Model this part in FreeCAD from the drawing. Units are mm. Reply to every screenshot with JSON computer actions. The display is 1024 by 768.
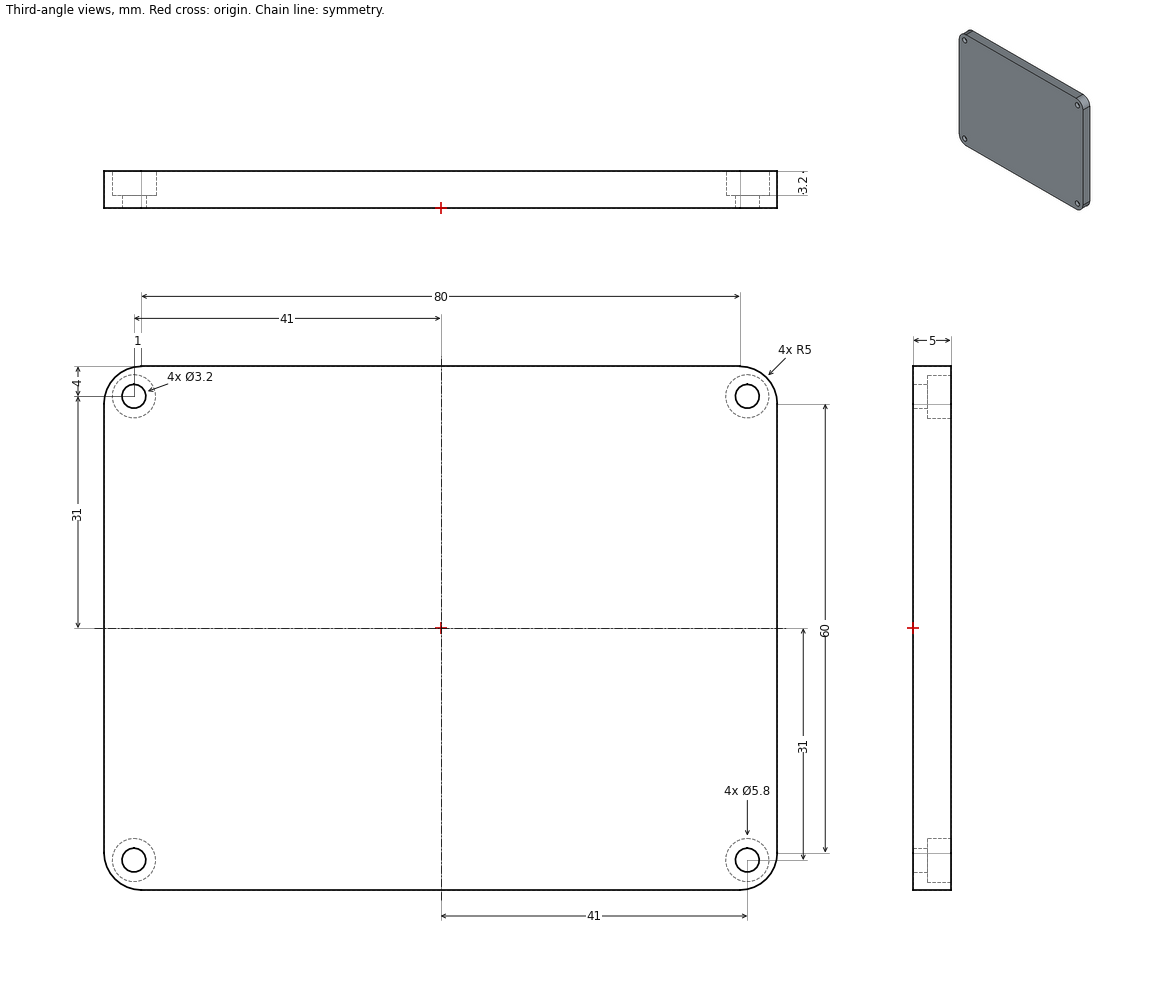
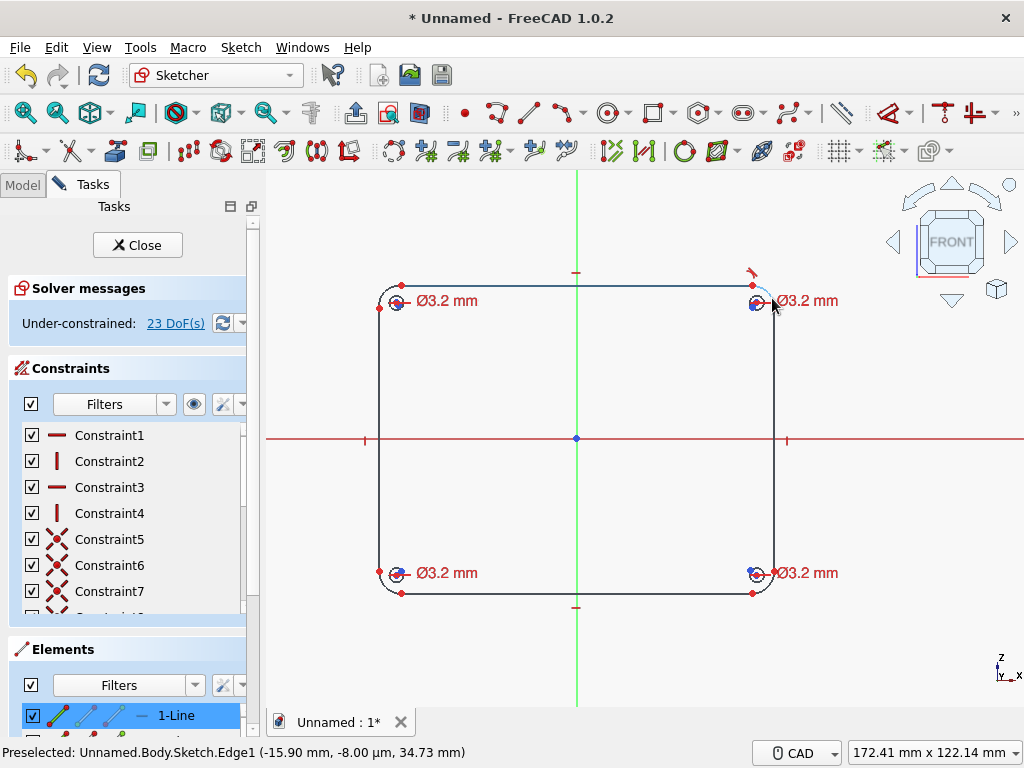
{"action": "scroll", "coordinate": [391, 288], "scroll_direction": "up", "scroll_amount": 2}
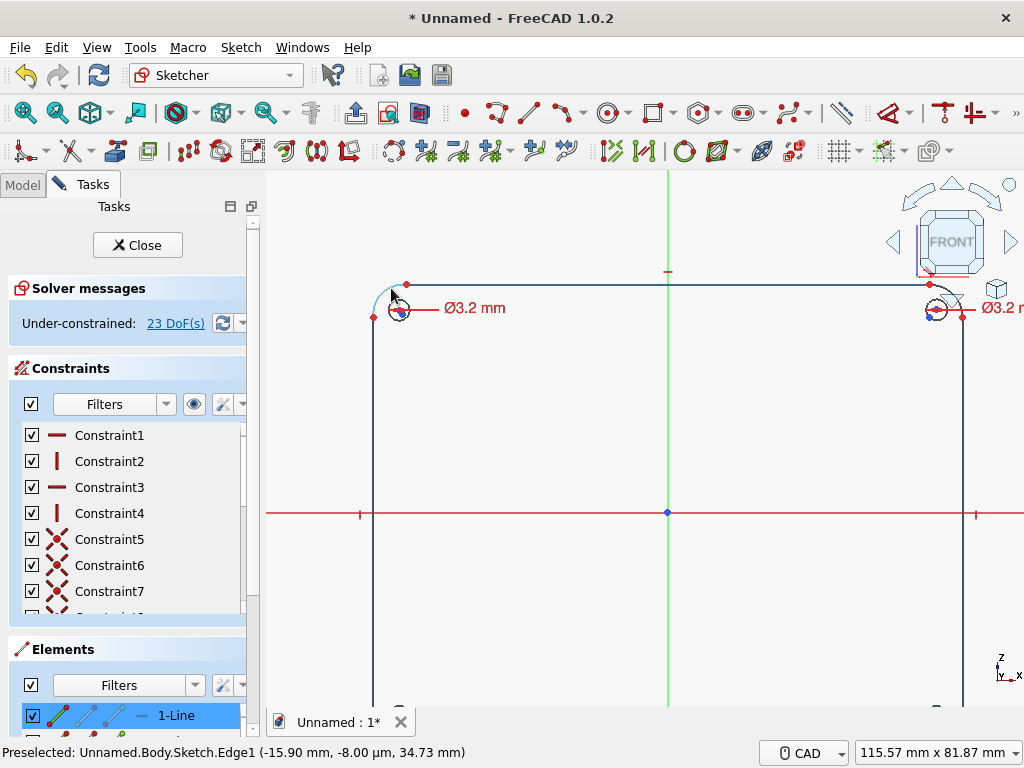
{"action": "left_click", "coordinate": [391, 287]}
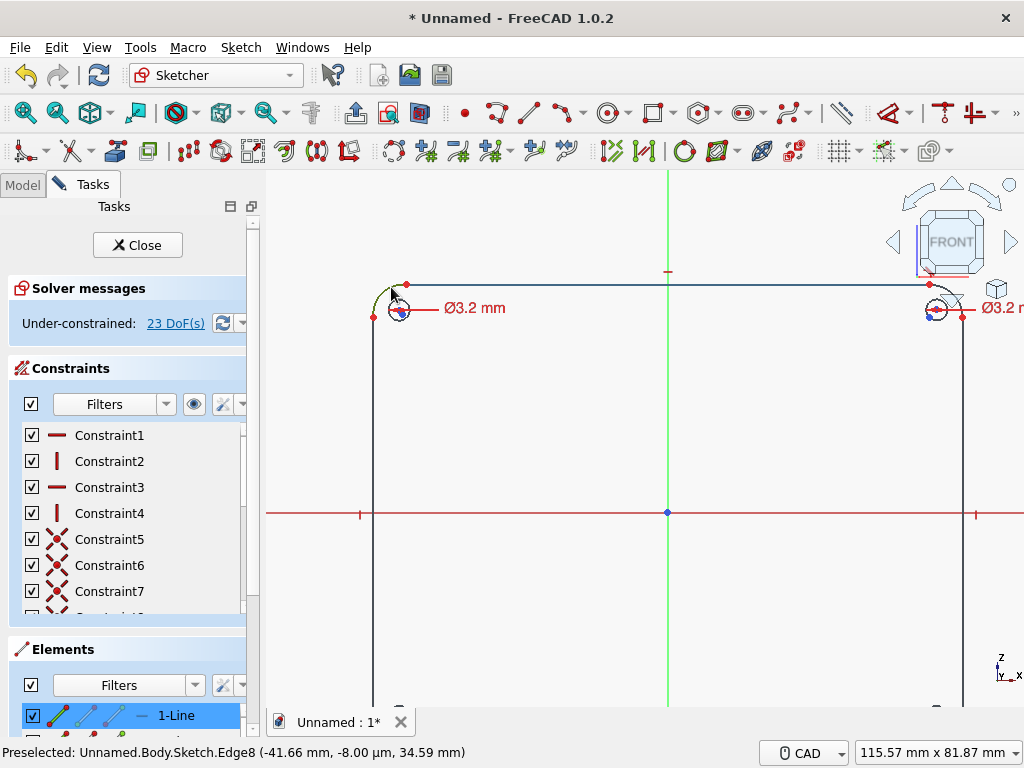
{"action": "key", "text": "t"}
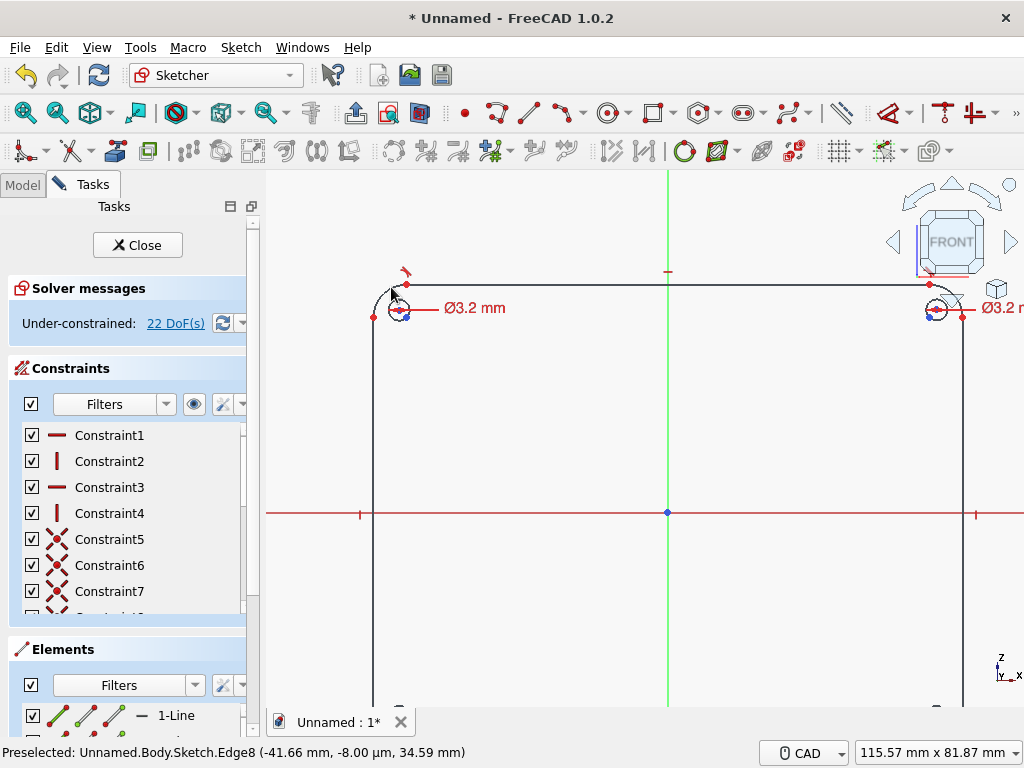
{"action": "scroll", "coordinate": [391, 288], "scroll_direction": "down", "scroll_amount": 2}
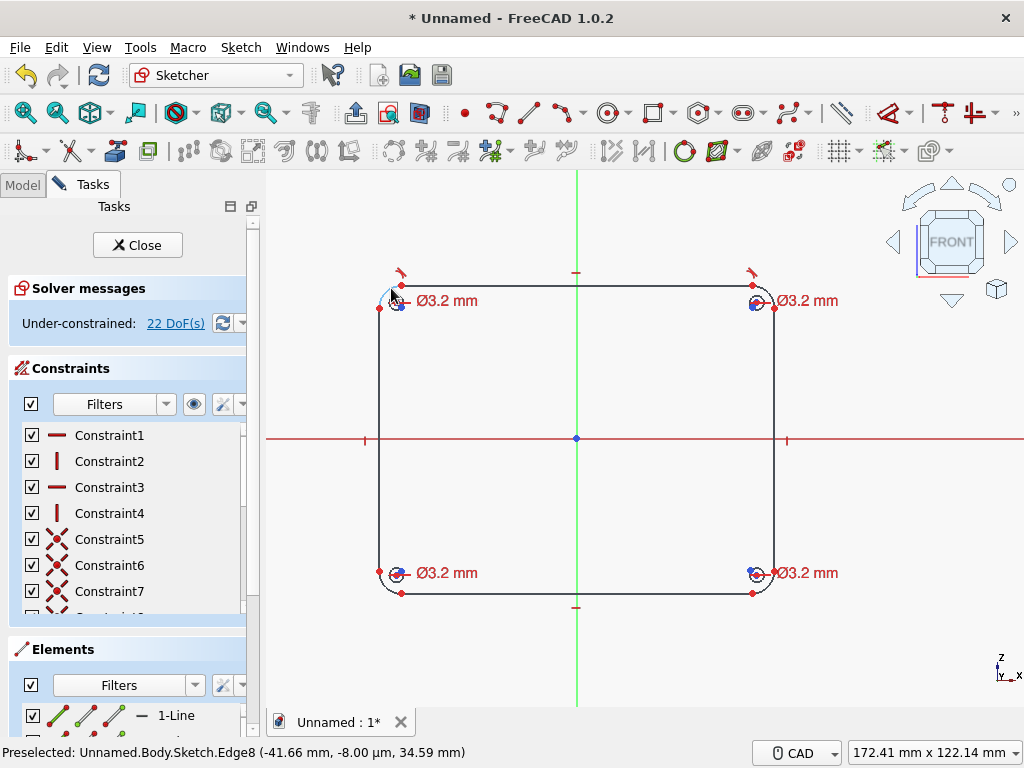
{"action": "left_click", "coordinate": [774, 387]}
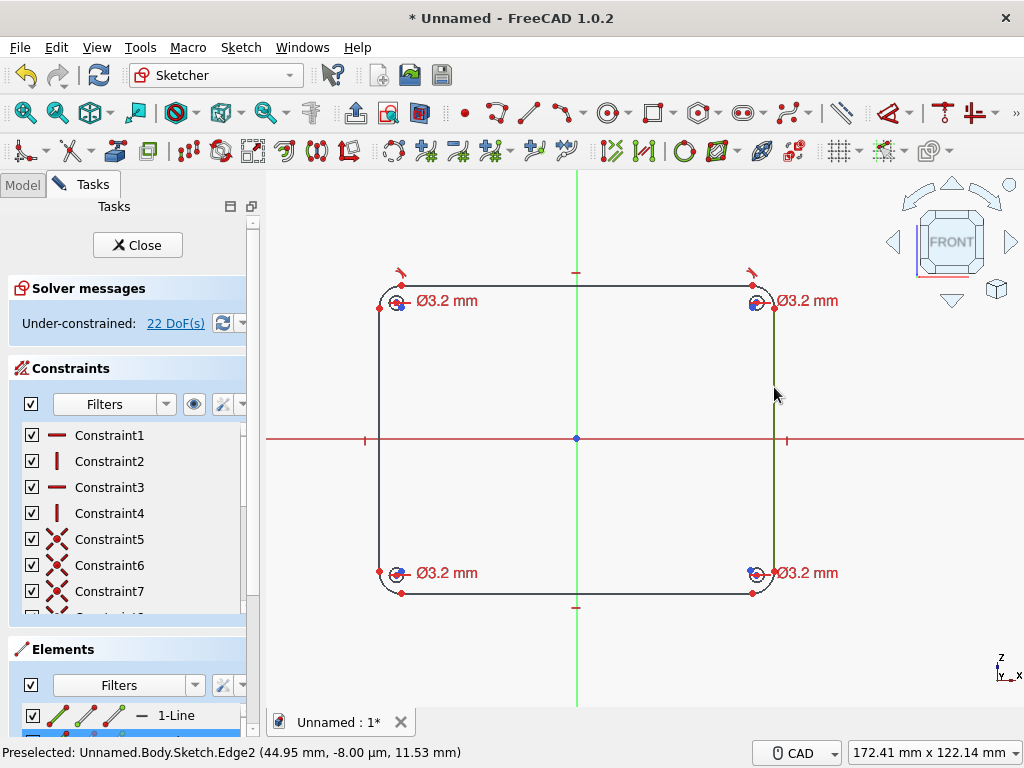
{"action": "scroll", "coordinate": [772, 298], "scroll_direction": "up", "scroll_amount": 3}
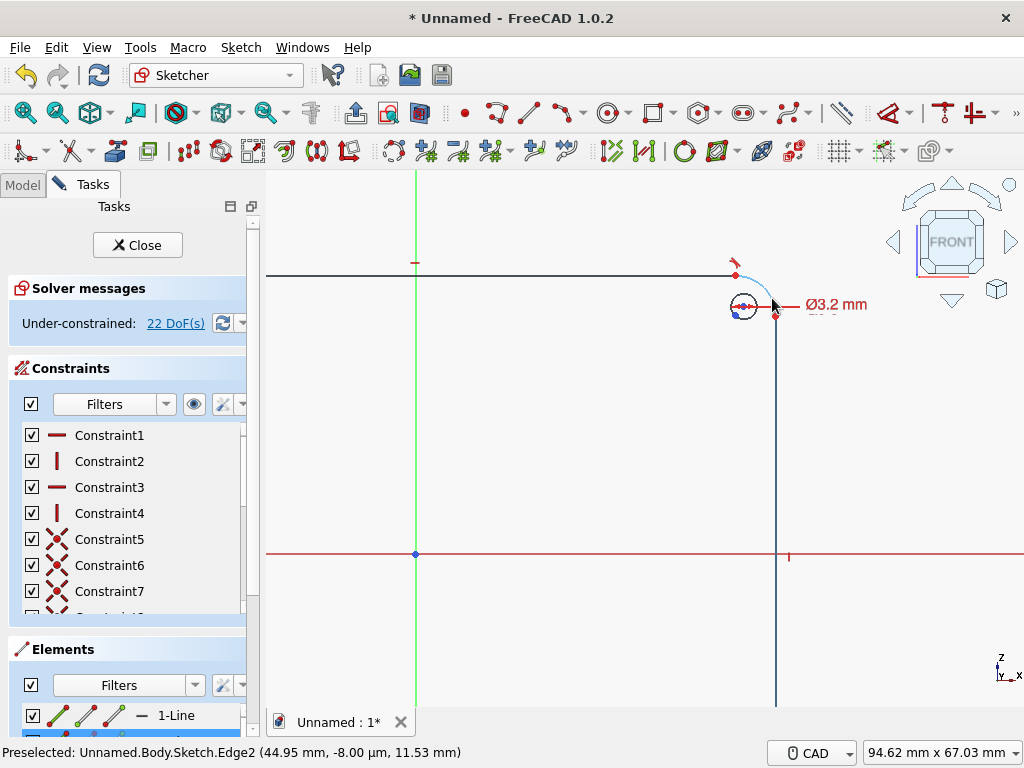
{"action": "left_click", "coordinate": [771, 298]}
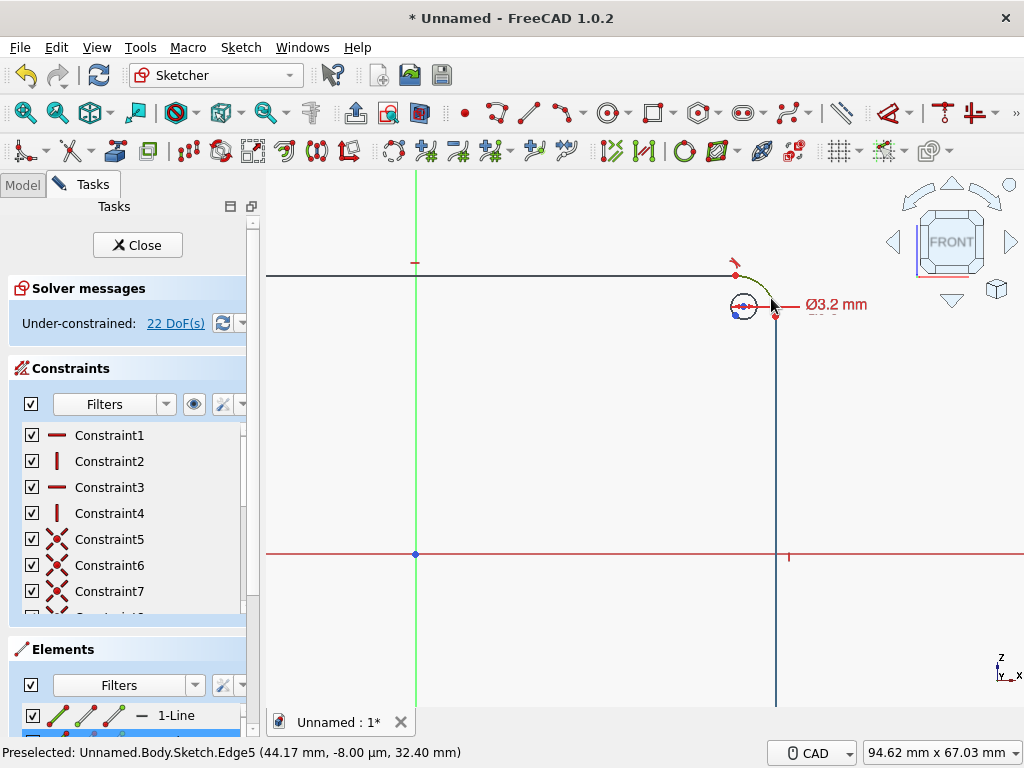
{"action": "key", "text": "t"}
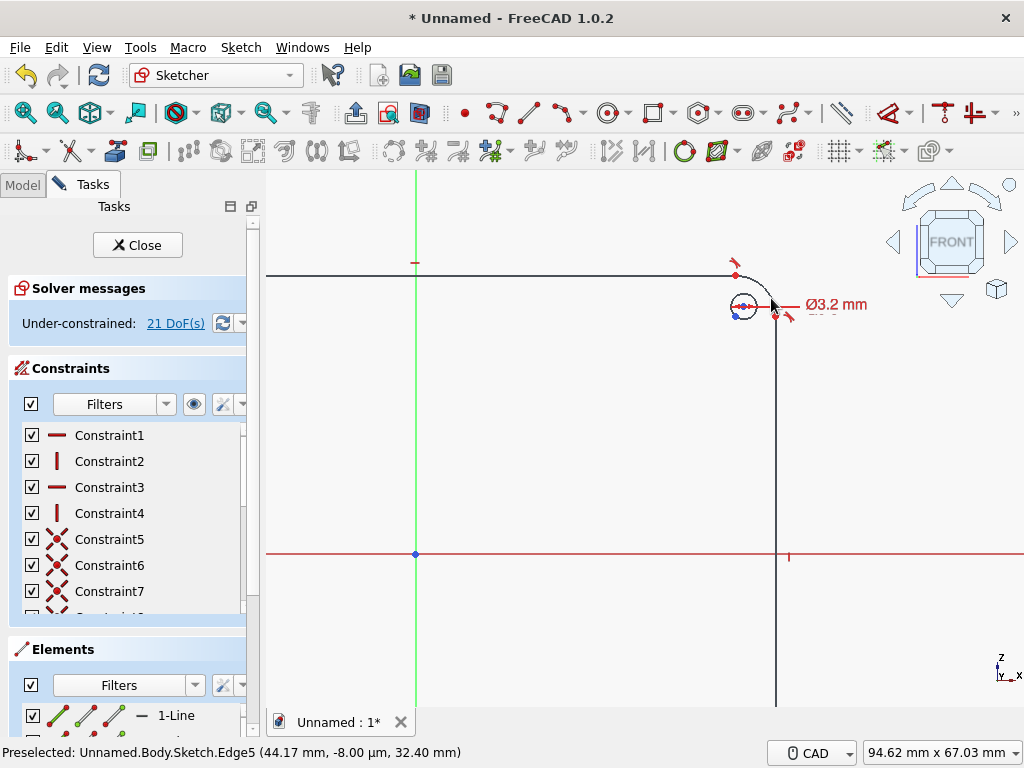
{"action": "left_click", "coordinate": [776, 460]}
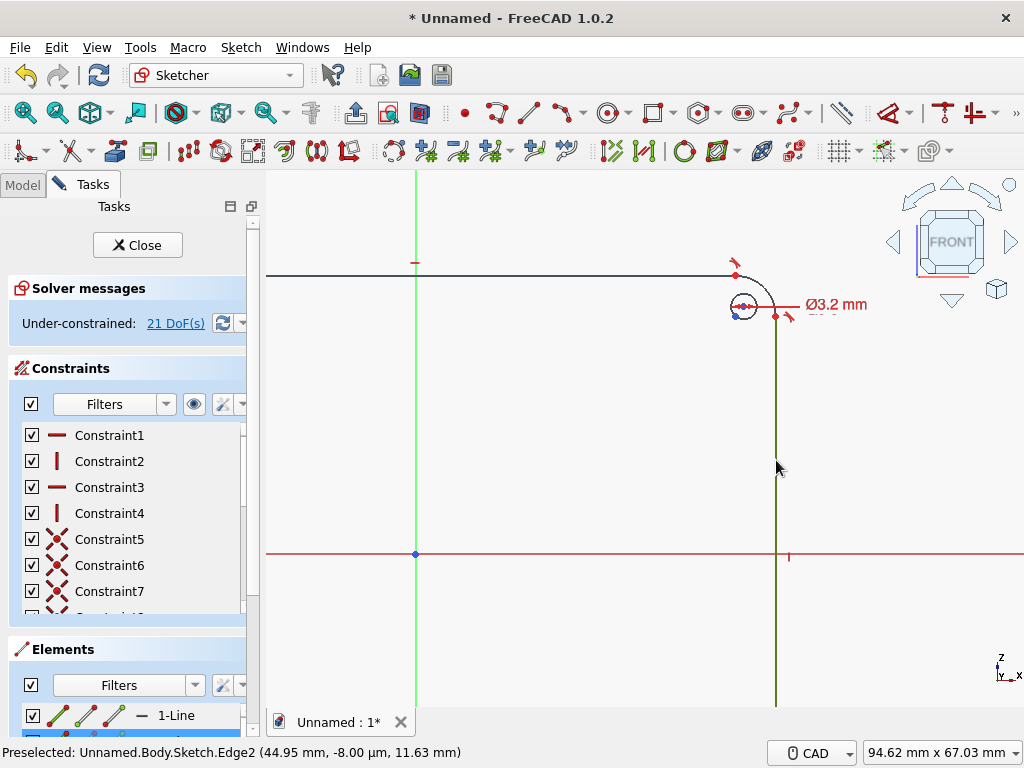
{"action": "scroll", "coordinate": [772, 298], "scroll_direction": "down", "scroll_amount": 3}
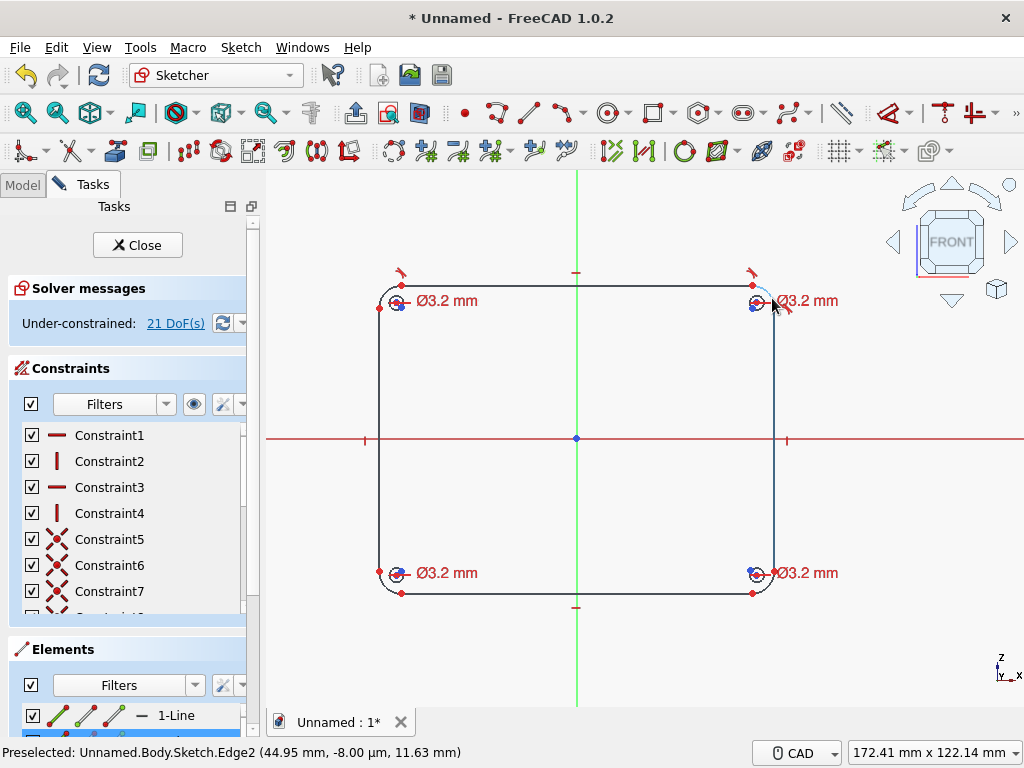
{"action": "scroll", "coordinate": [762, 591], "scroll_direction": "up", "scroll_amount": 2}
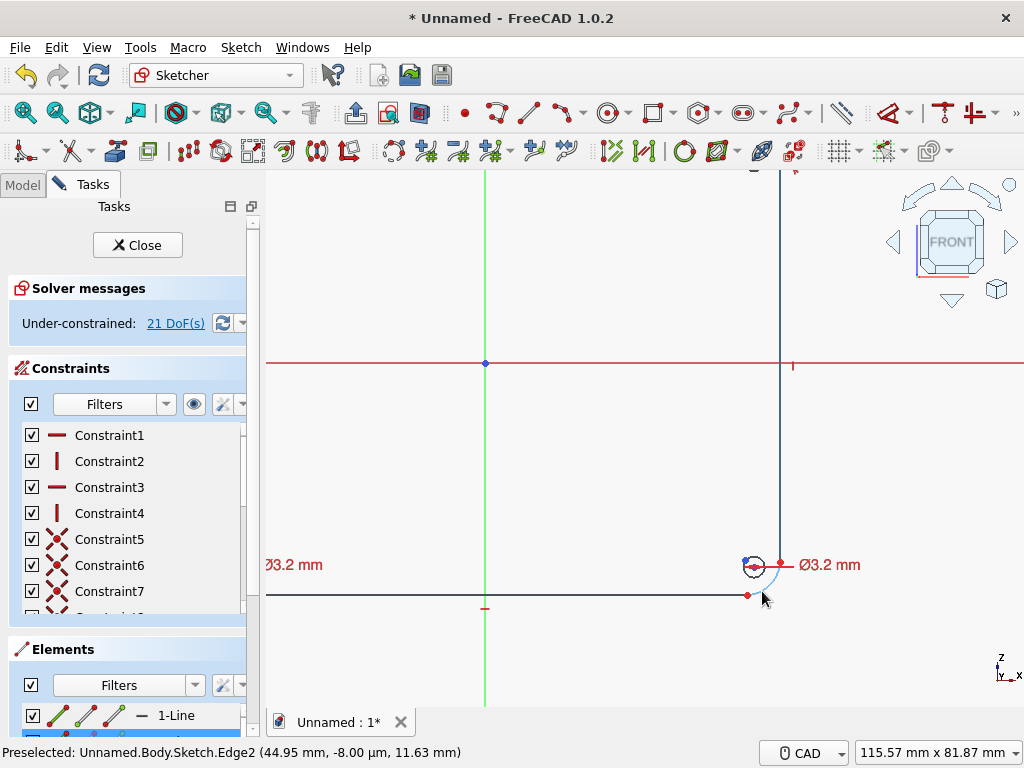
{"action": "left_click", "coordinate": [762, 591]}